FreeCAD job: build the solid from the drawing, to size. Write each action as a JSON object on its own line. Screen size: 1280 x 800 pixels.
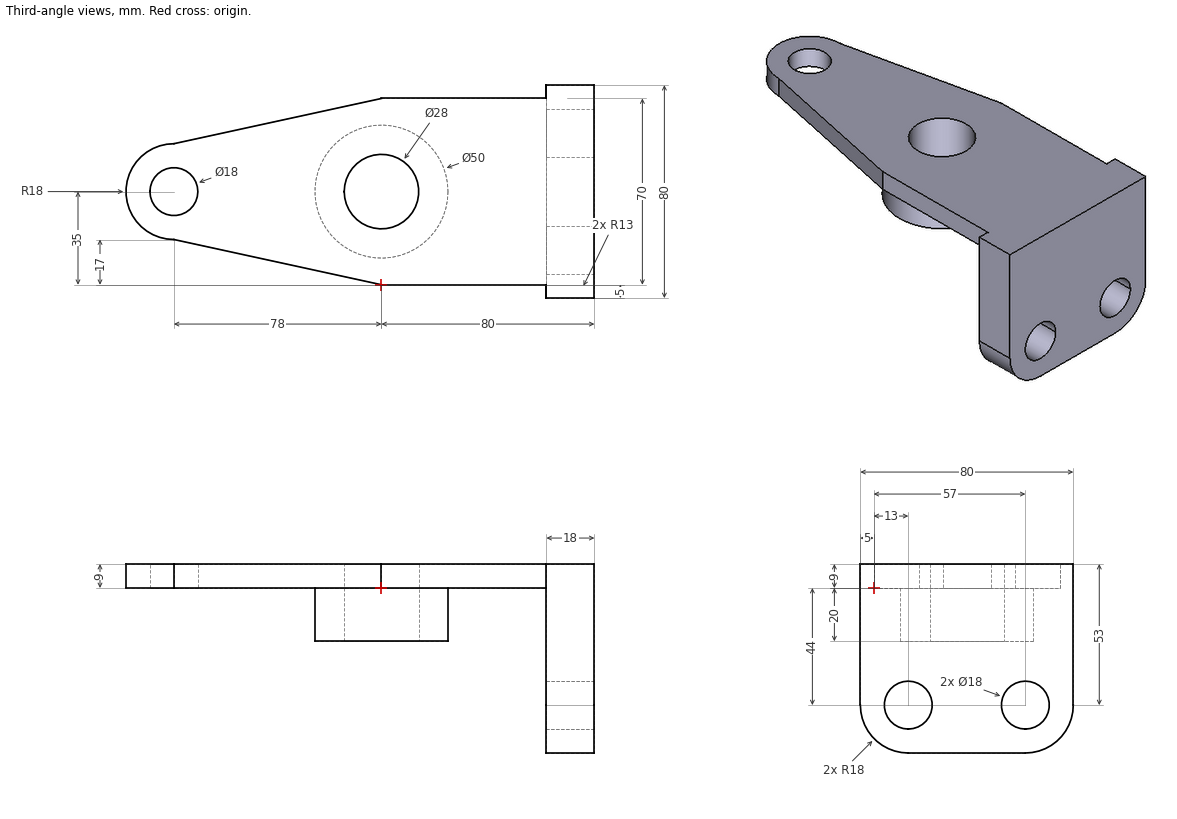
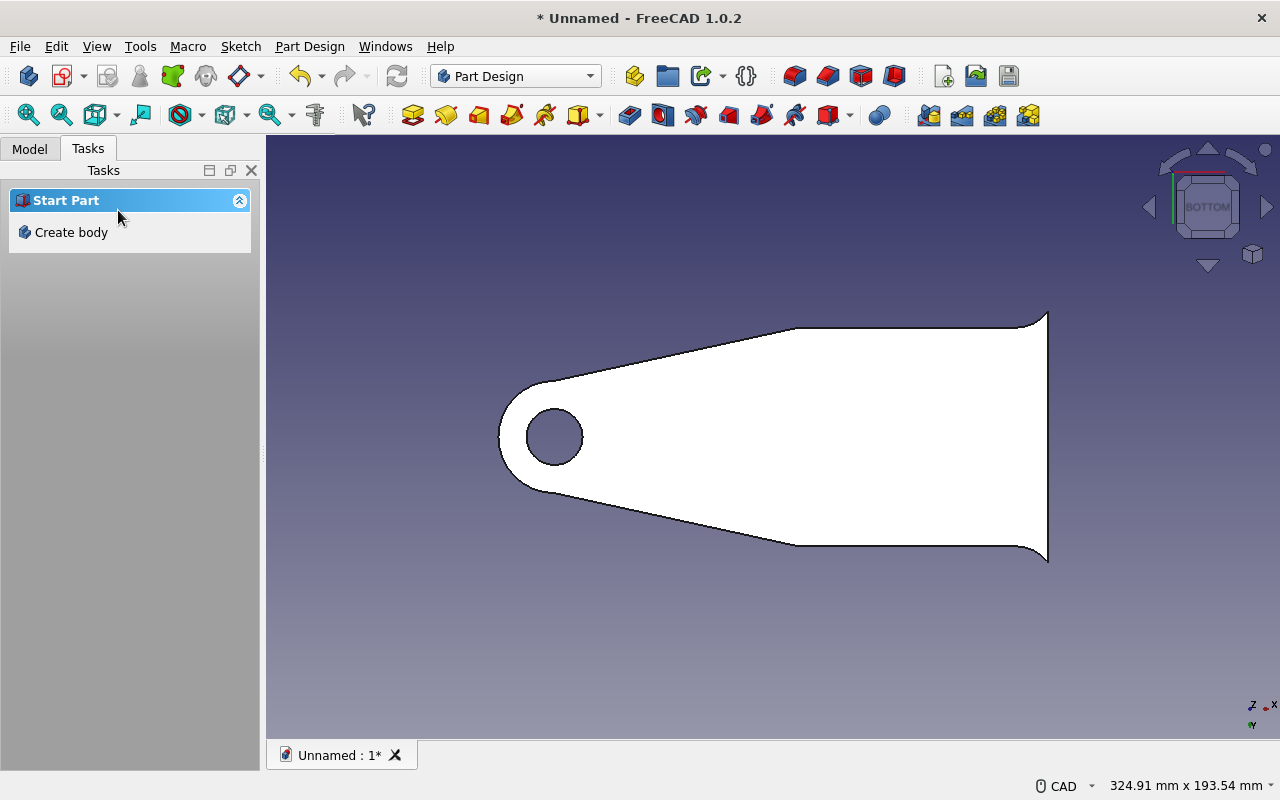
{"action": "left_click", "coordinate": [930, 436]}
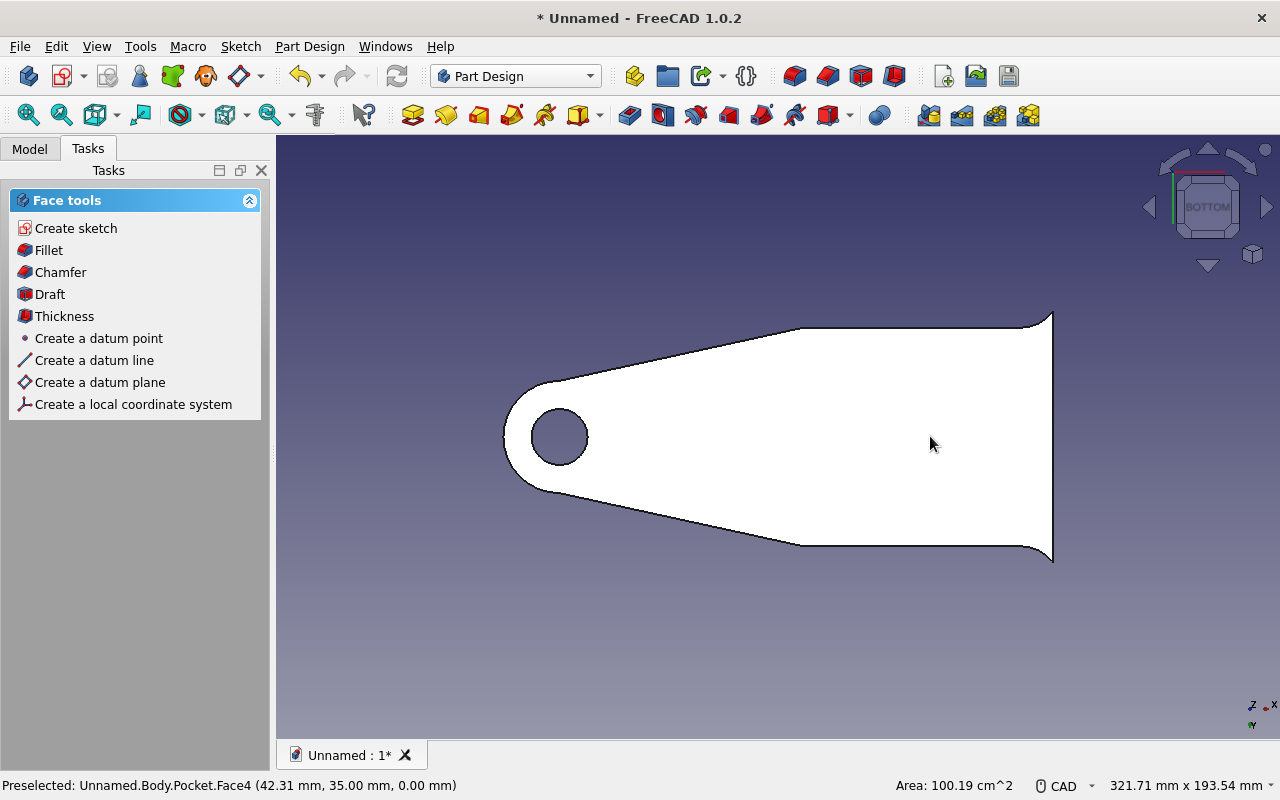
{"action": "left_click", "coordinate": [62, 76]}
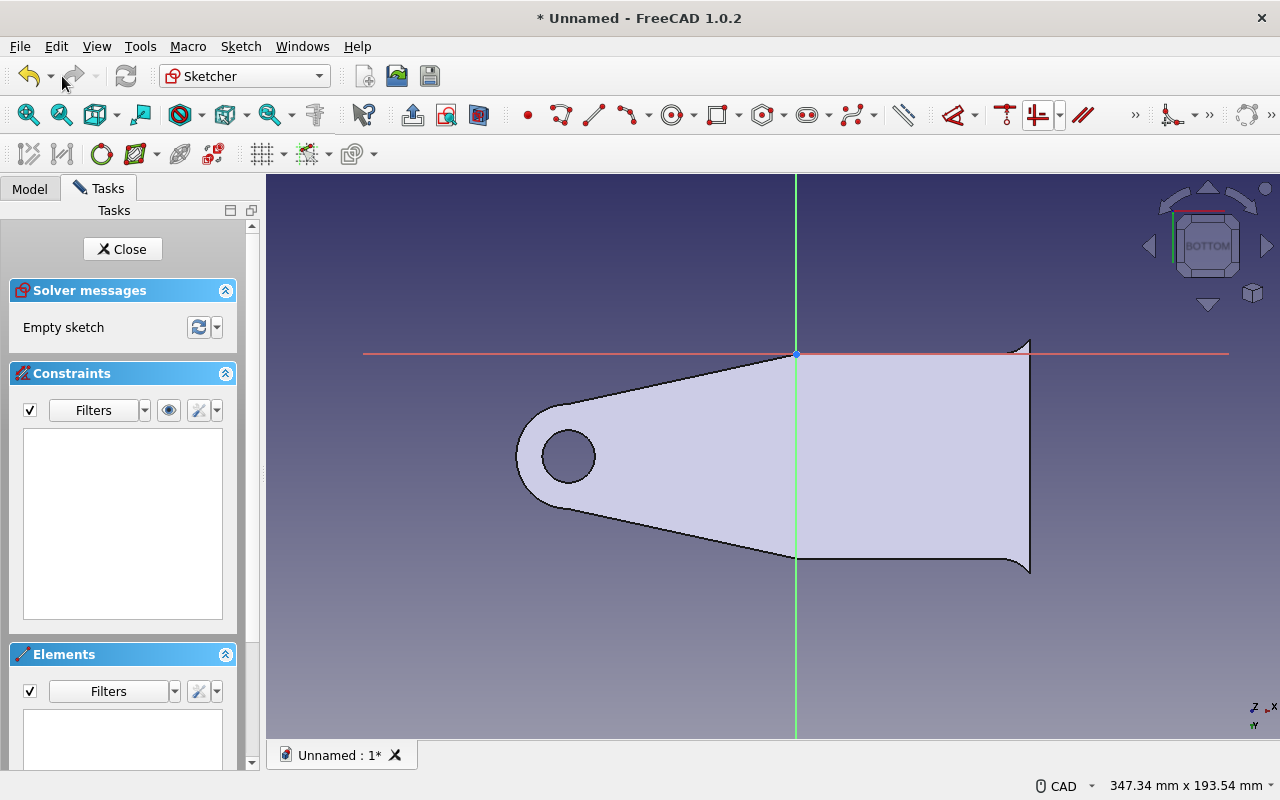
{"action": "scroll", "coordinate": [871, 430], "scroll_direction": "up", "scroll_amount": 4}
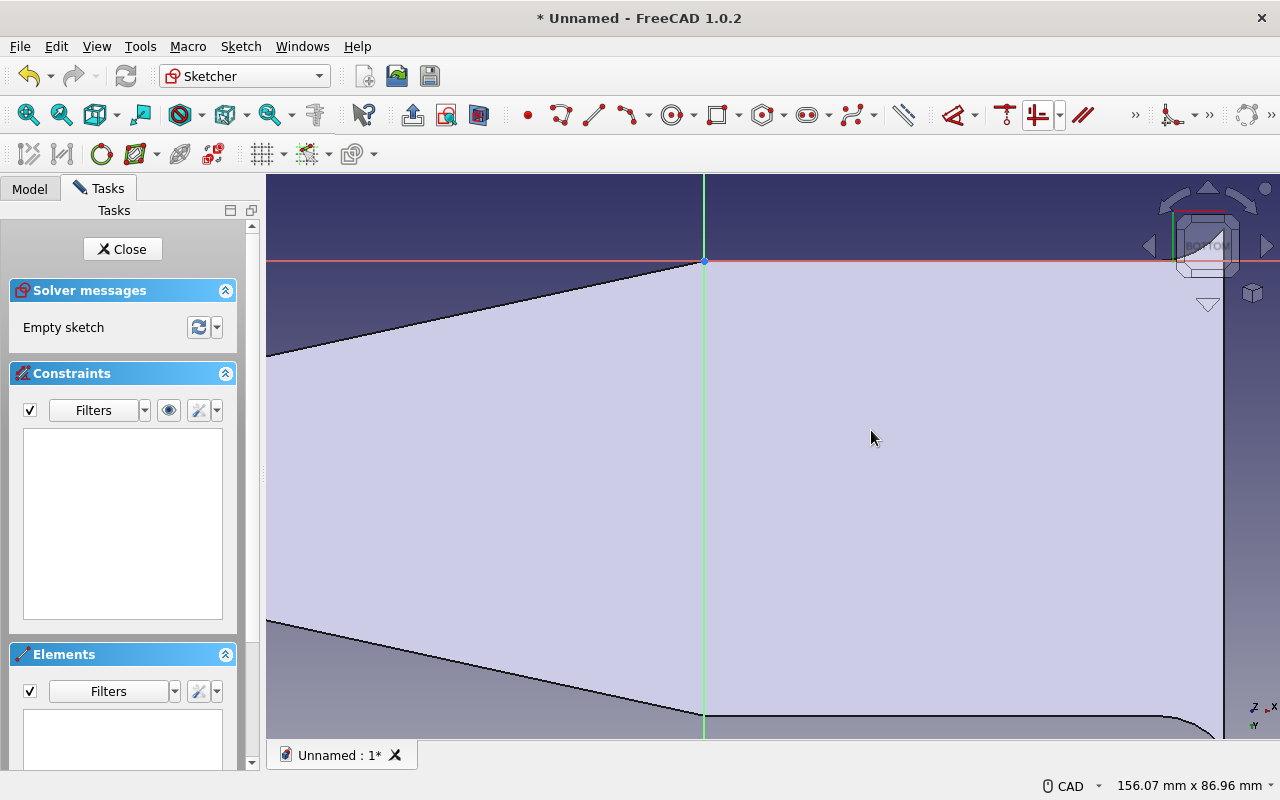
{"action": "left_click", "coordinate": [672, 116]}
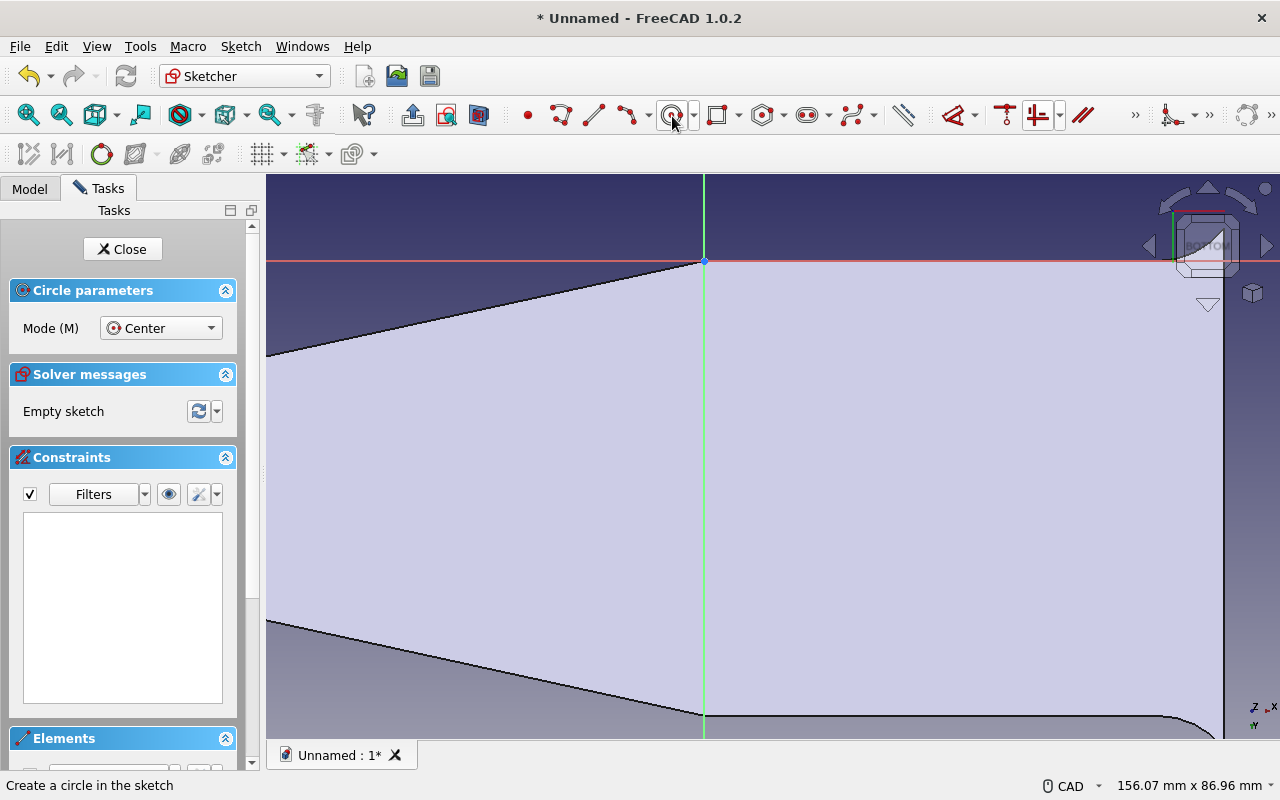
{"action": "left_click", "coordinate": [704, 488]}
{"action": "left_click", "coordinate": [819, 374]}
{"action": "key", "text": "Escape"}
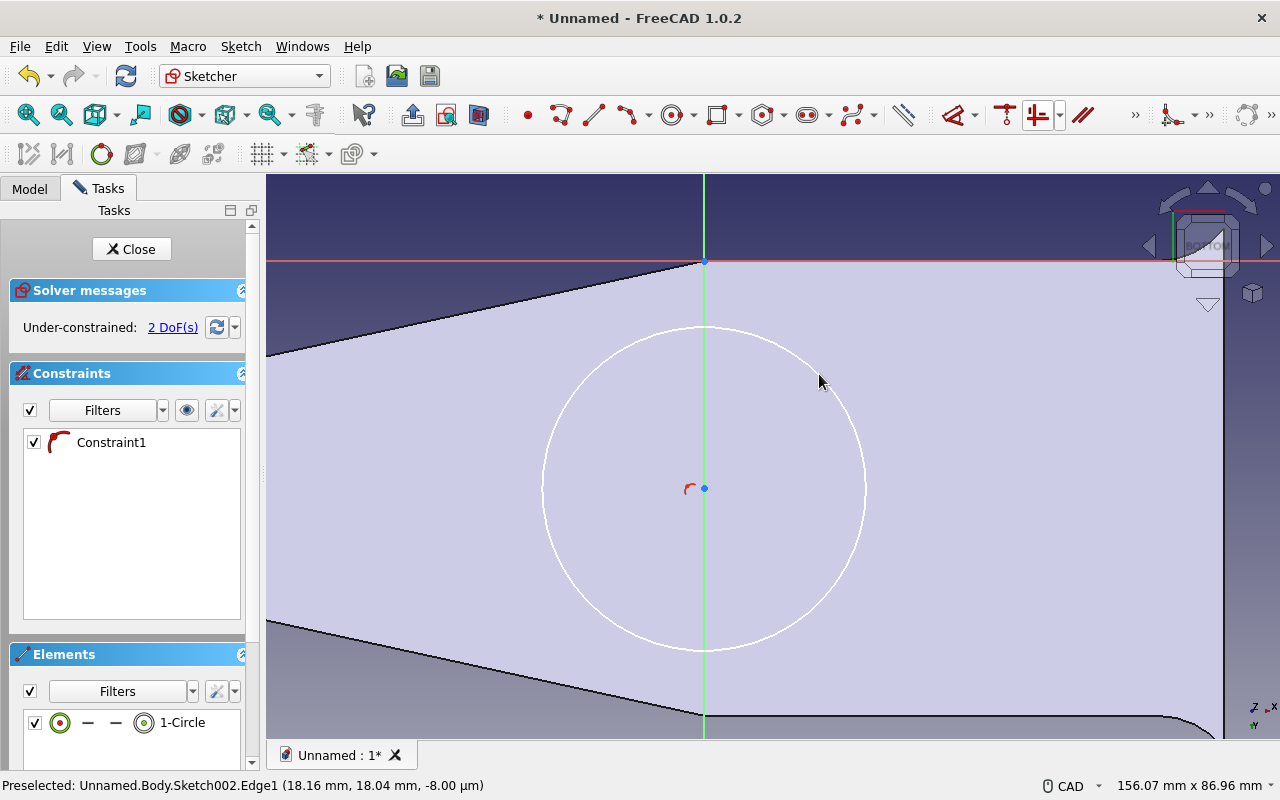
{"action": "left_click", "coordinate": [952, 116]}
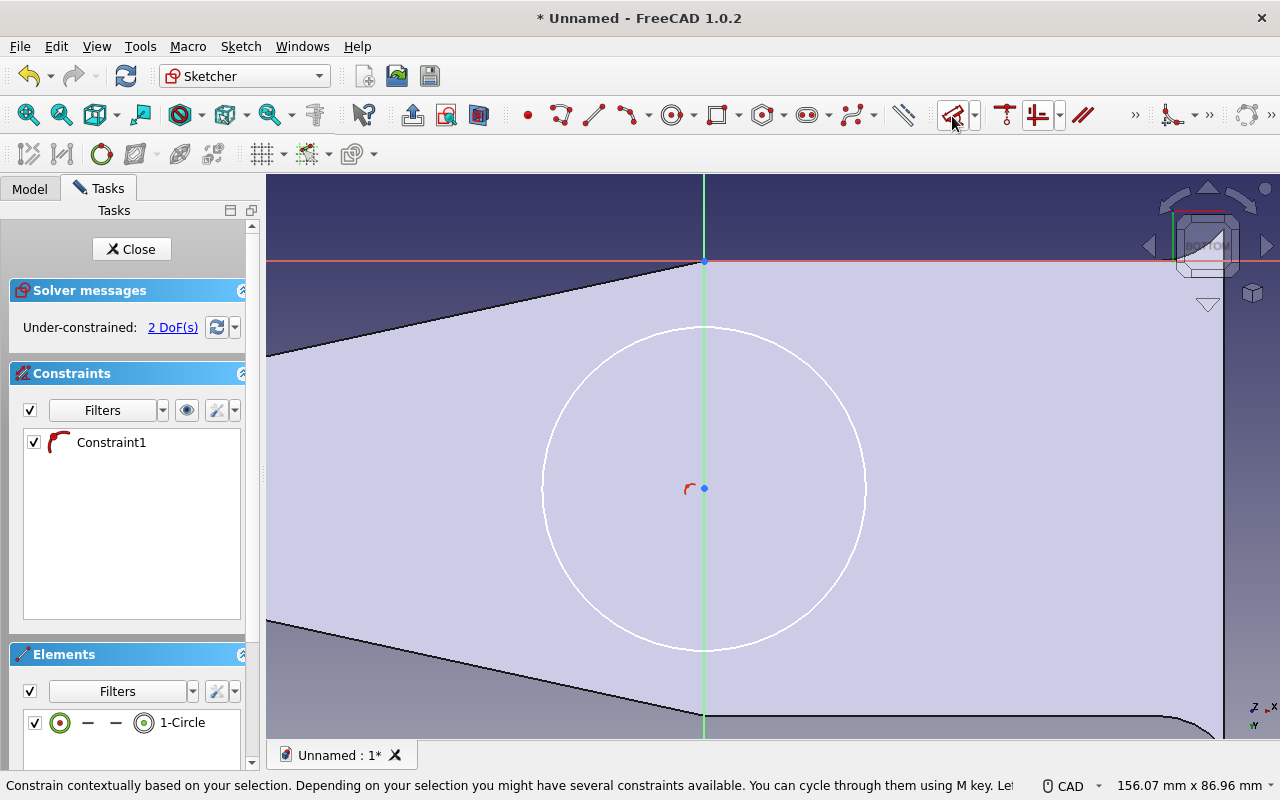
{"action": "left_click", "coordinate": [818, 374]}
{"action": "left_click", "coordinate": [841, 351]}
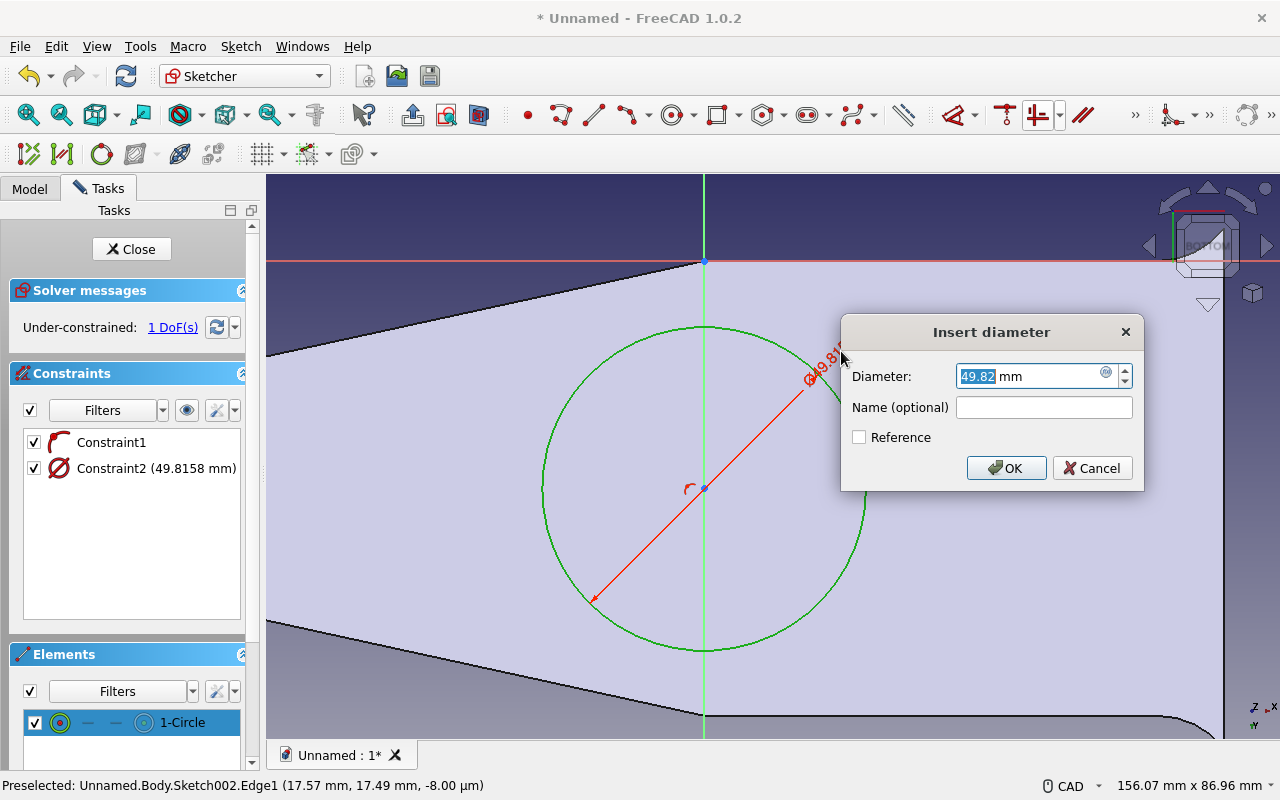
{"action": "type", "text": "50"}
{"action": "key", "text": "Return"}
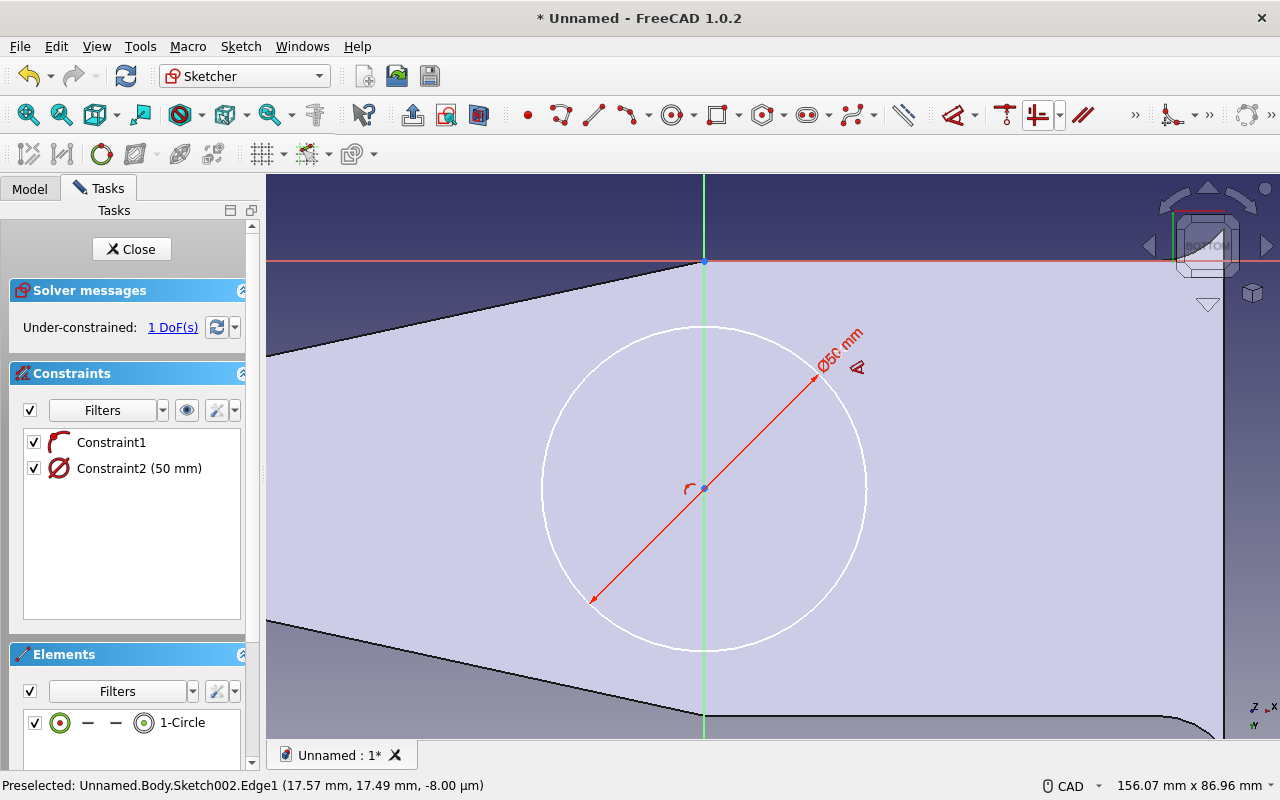
{"action": "left_click", "coordinate": [704, 489]}
{"action": "left_click", "coordinate": [738, 375]}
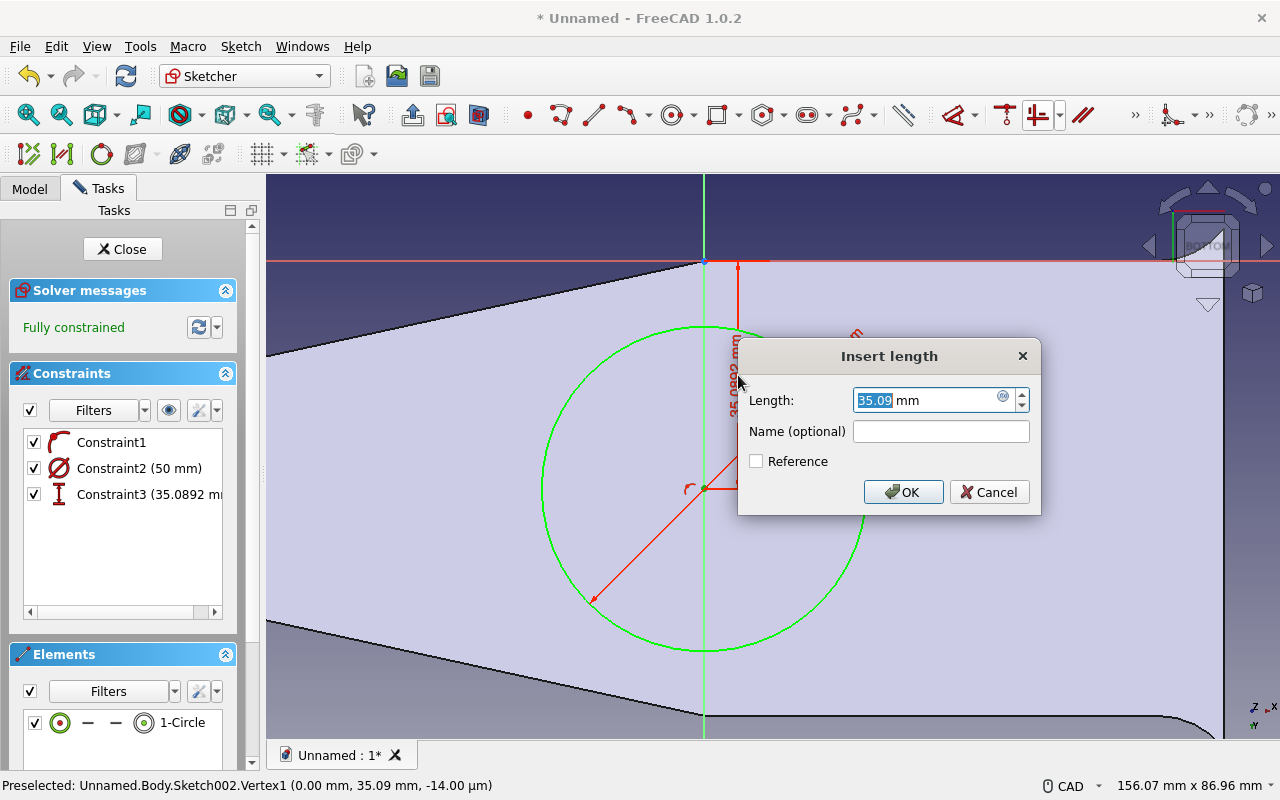
{"action": "type", "text": "35"}
{"action": "key", "text": "Return"}
{"action": "key", "text": "Escape"}